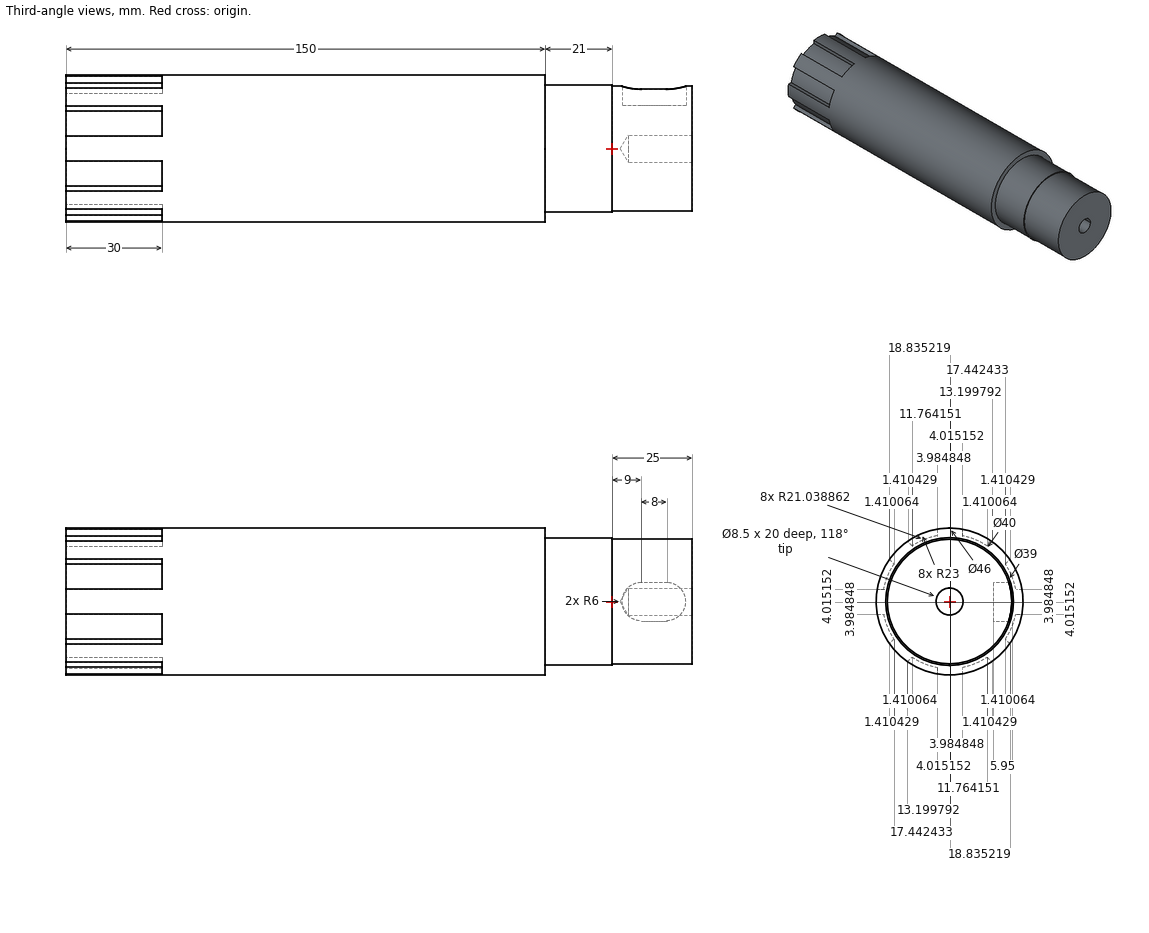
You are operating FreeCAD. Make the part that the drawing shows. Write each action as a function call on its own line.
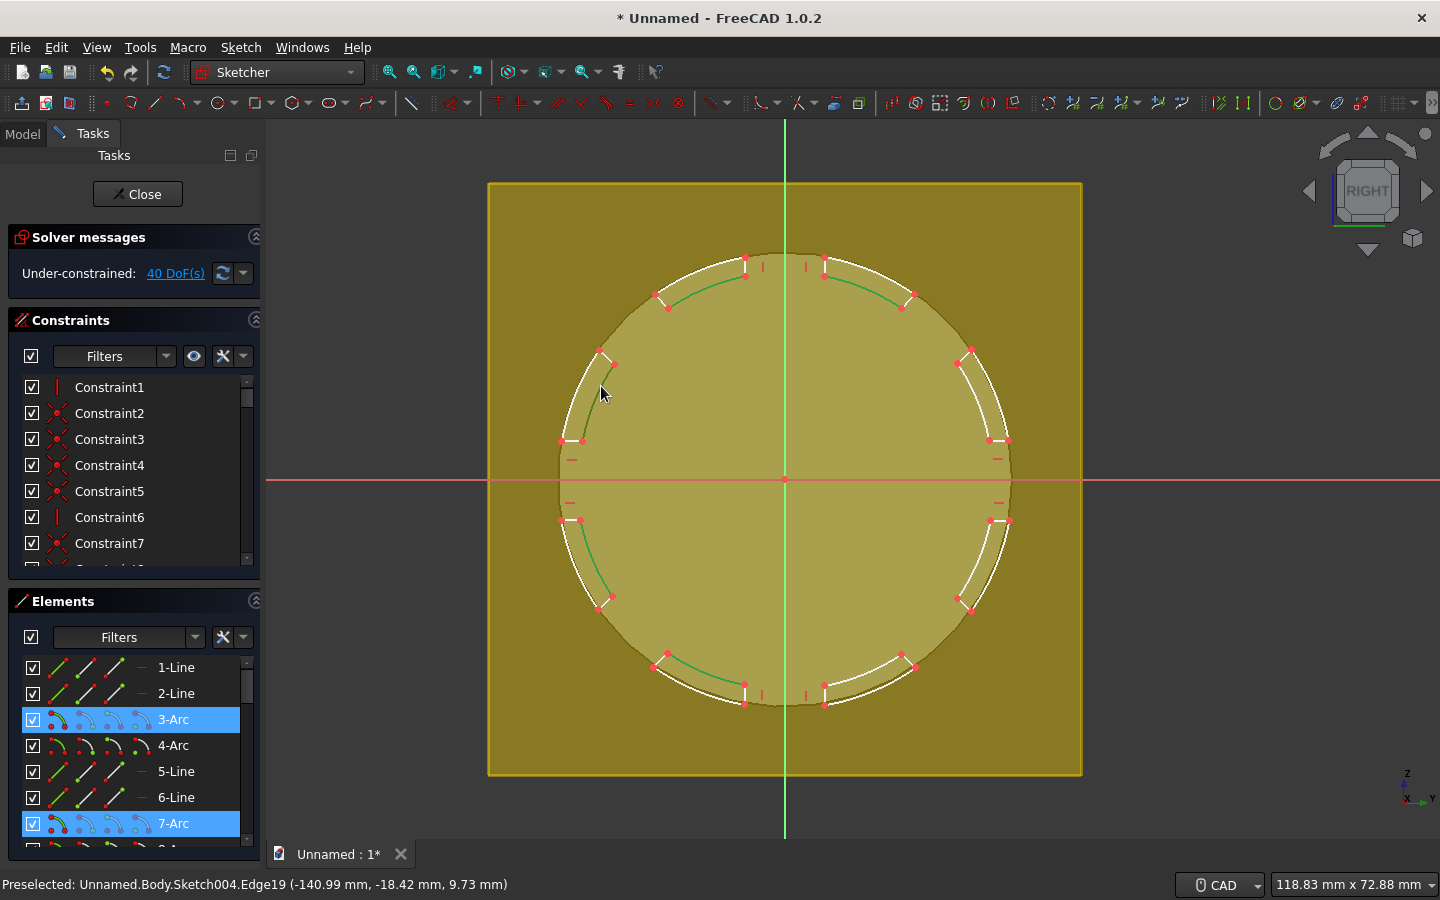
click(983, 416)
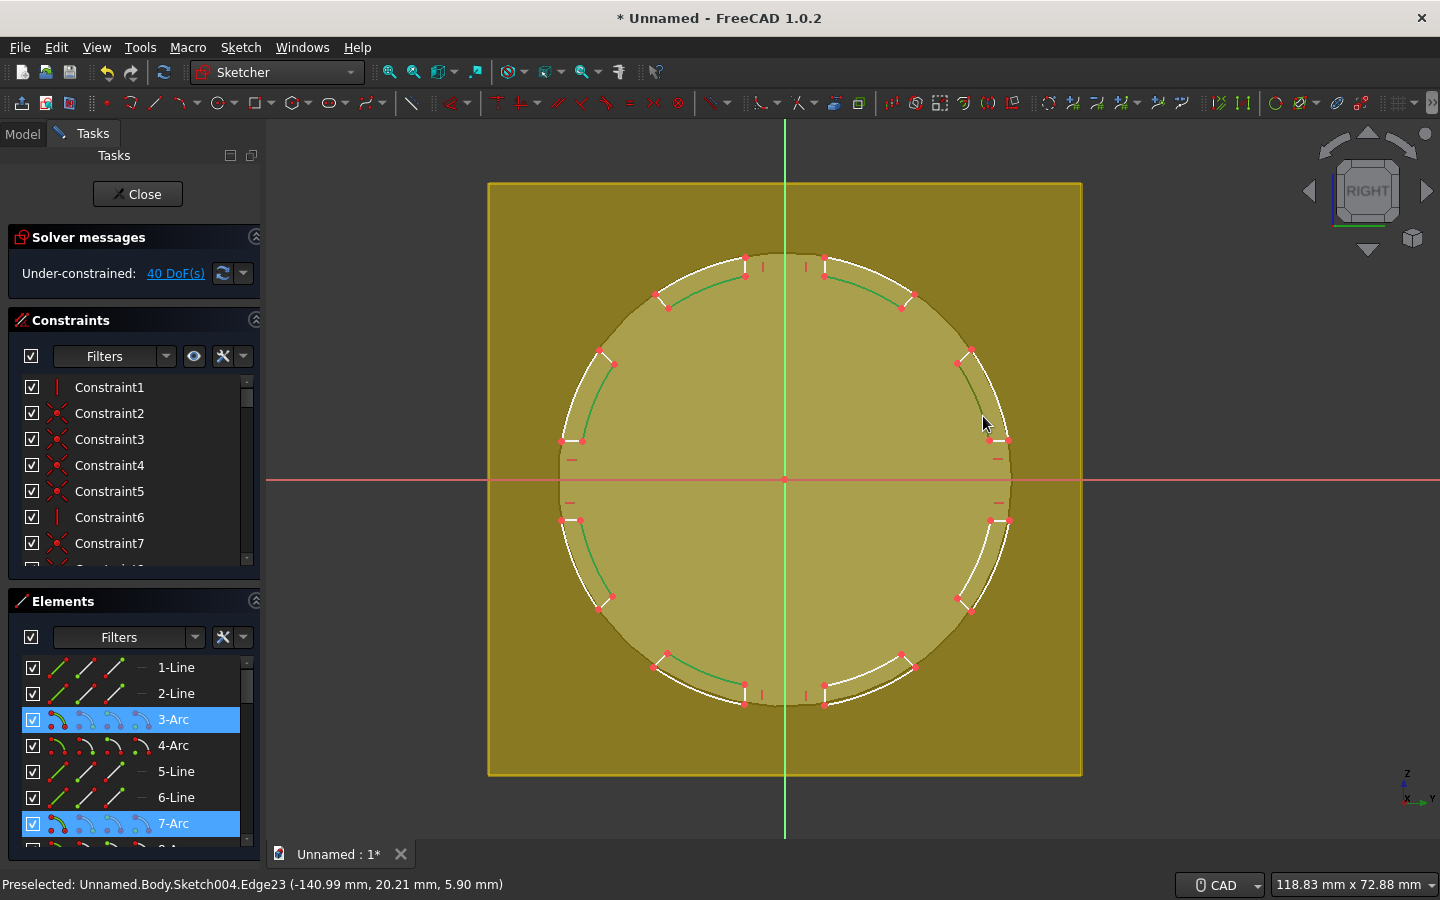
click(971, 576)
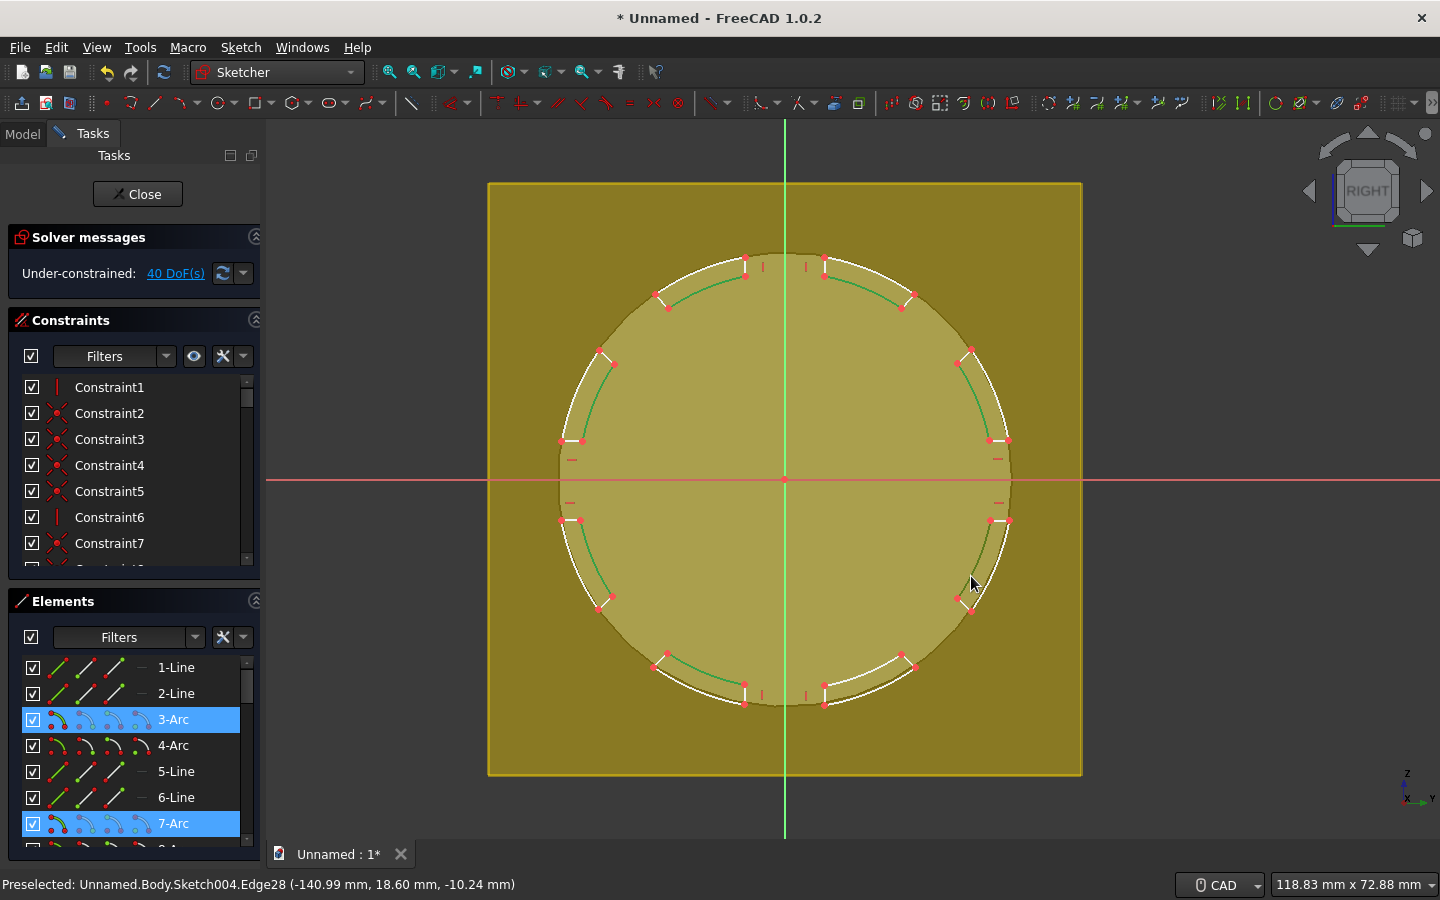
click(849, 680)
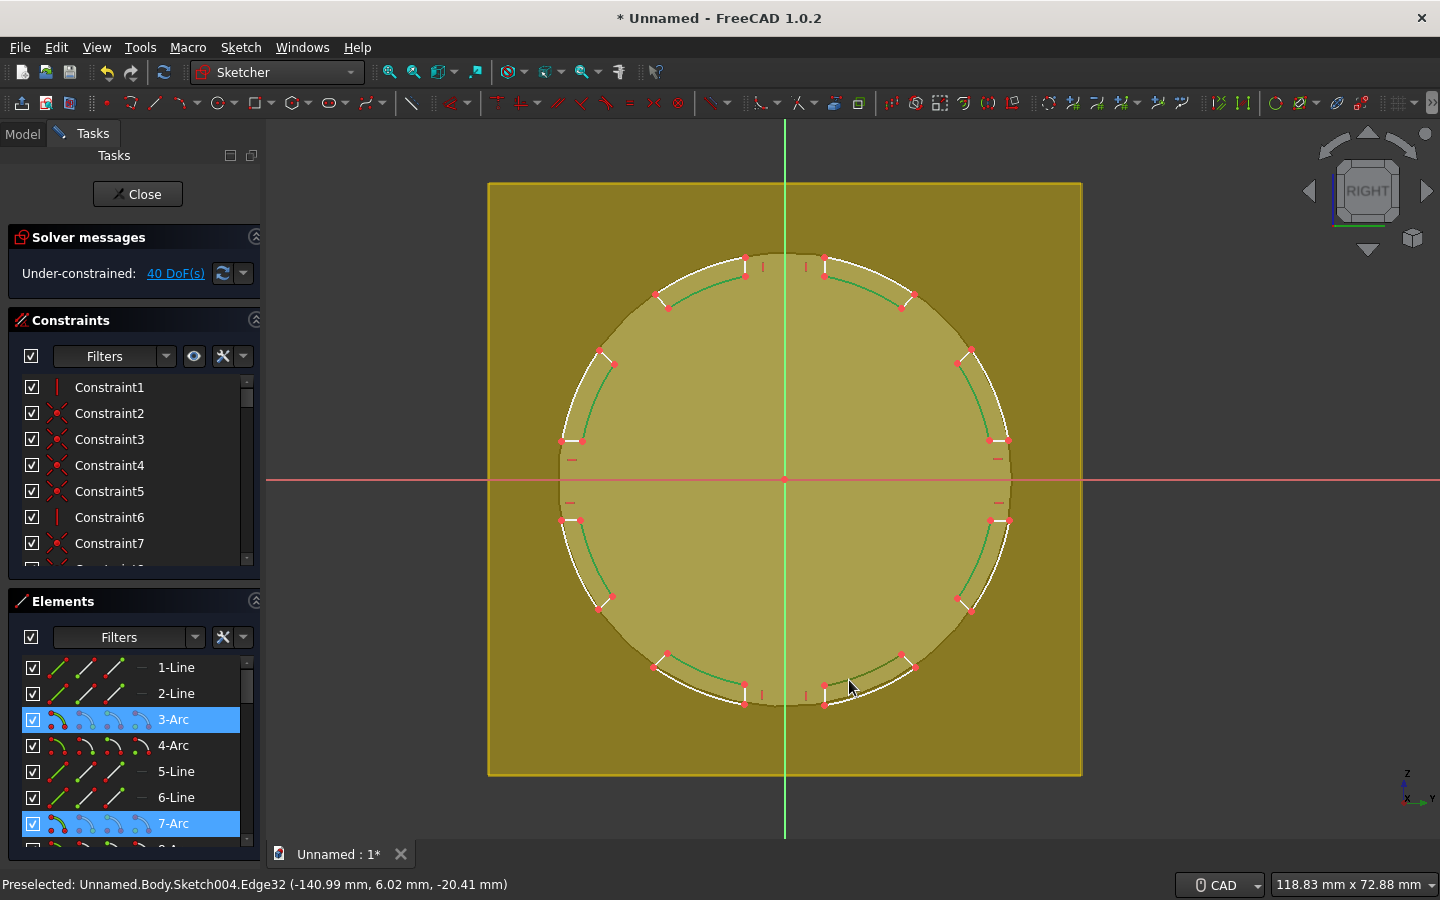
click(630, 104)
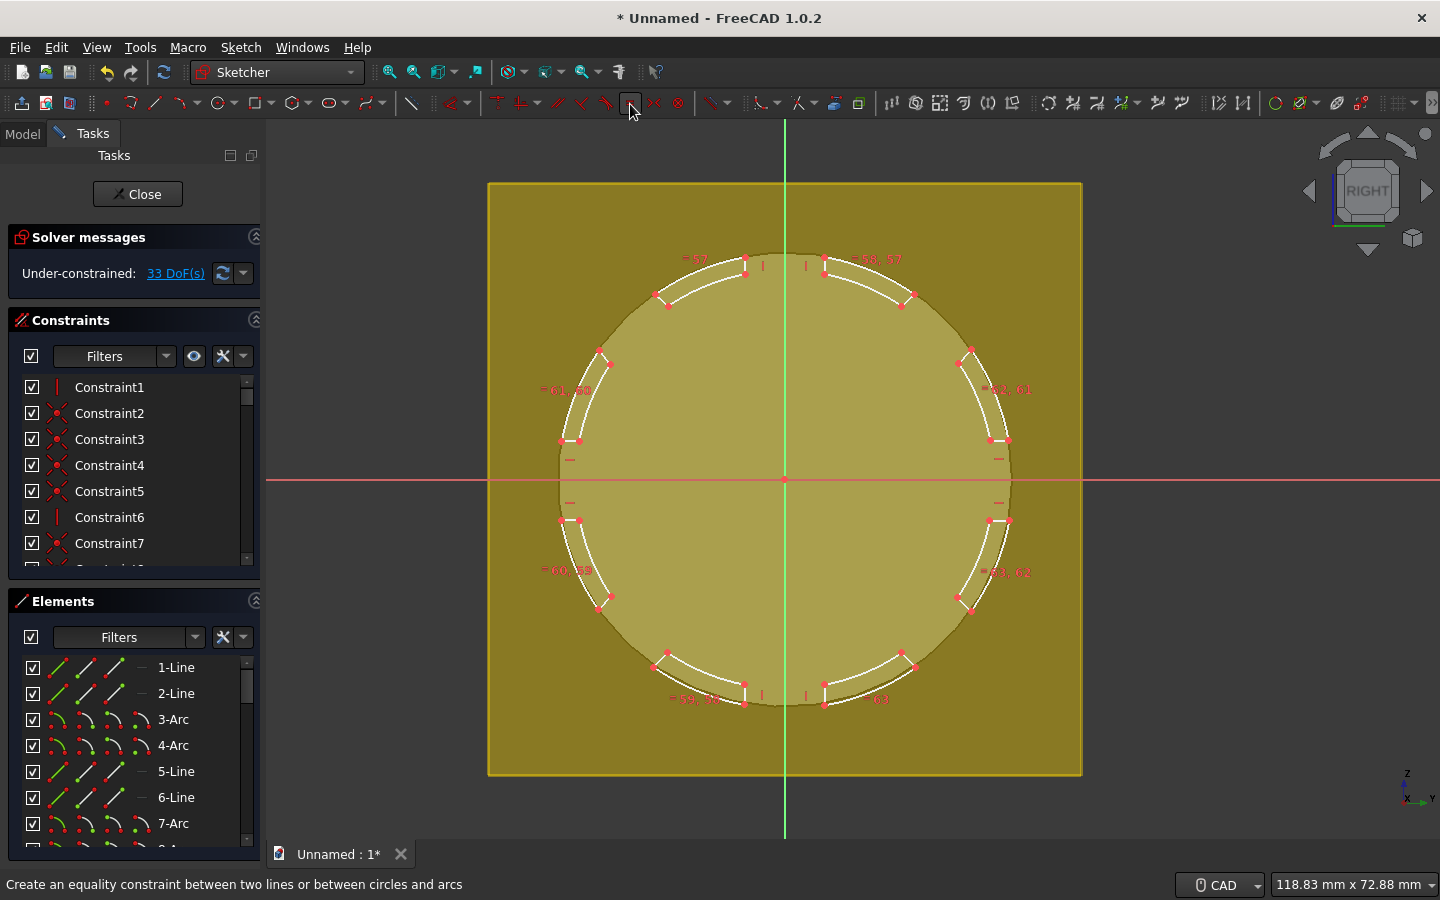
click(717, 264)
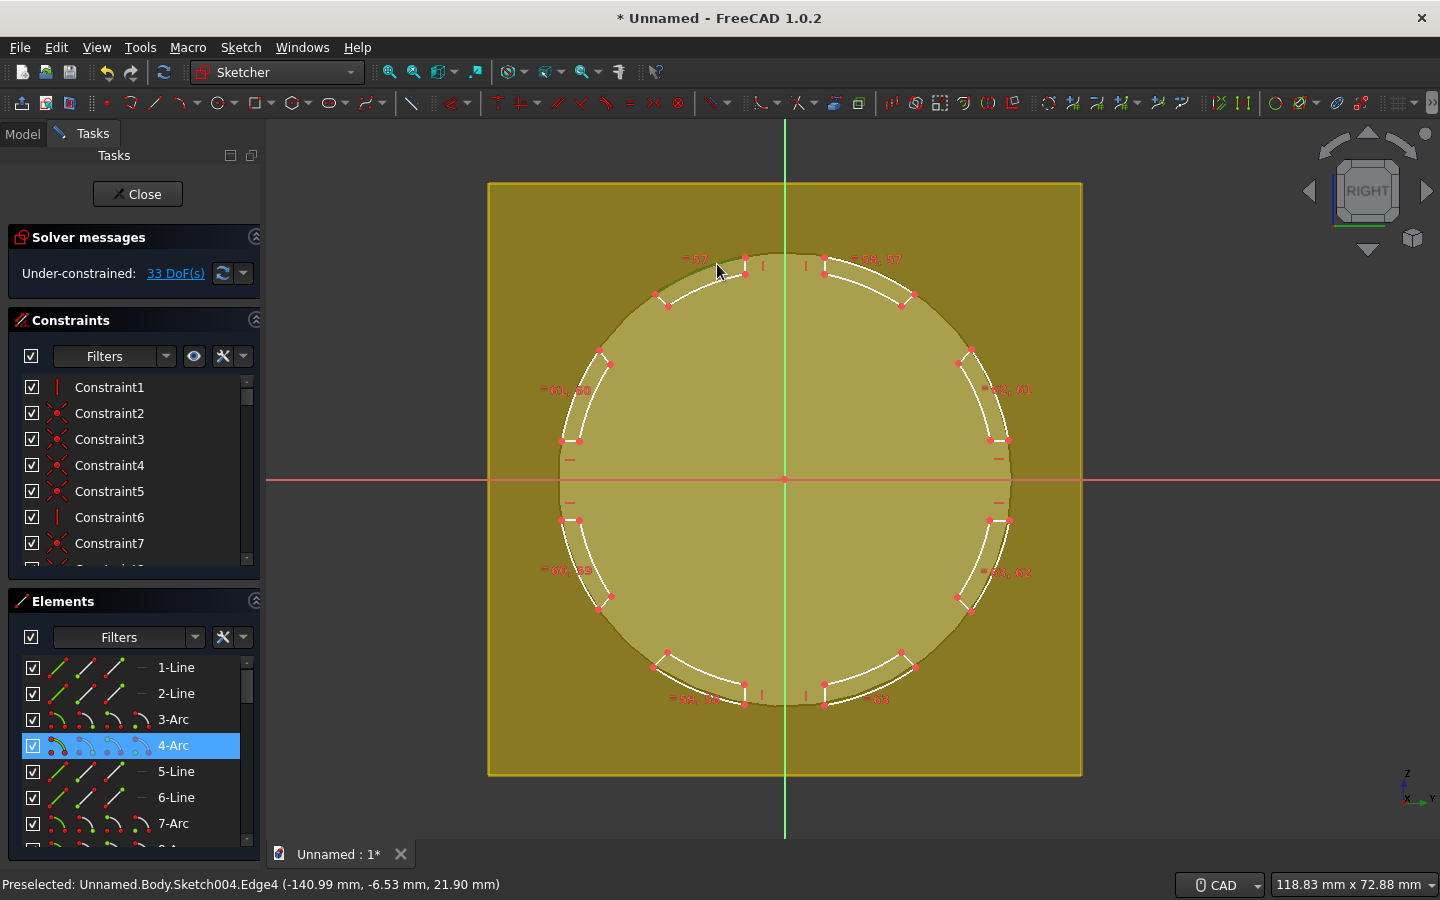
click(890, 279)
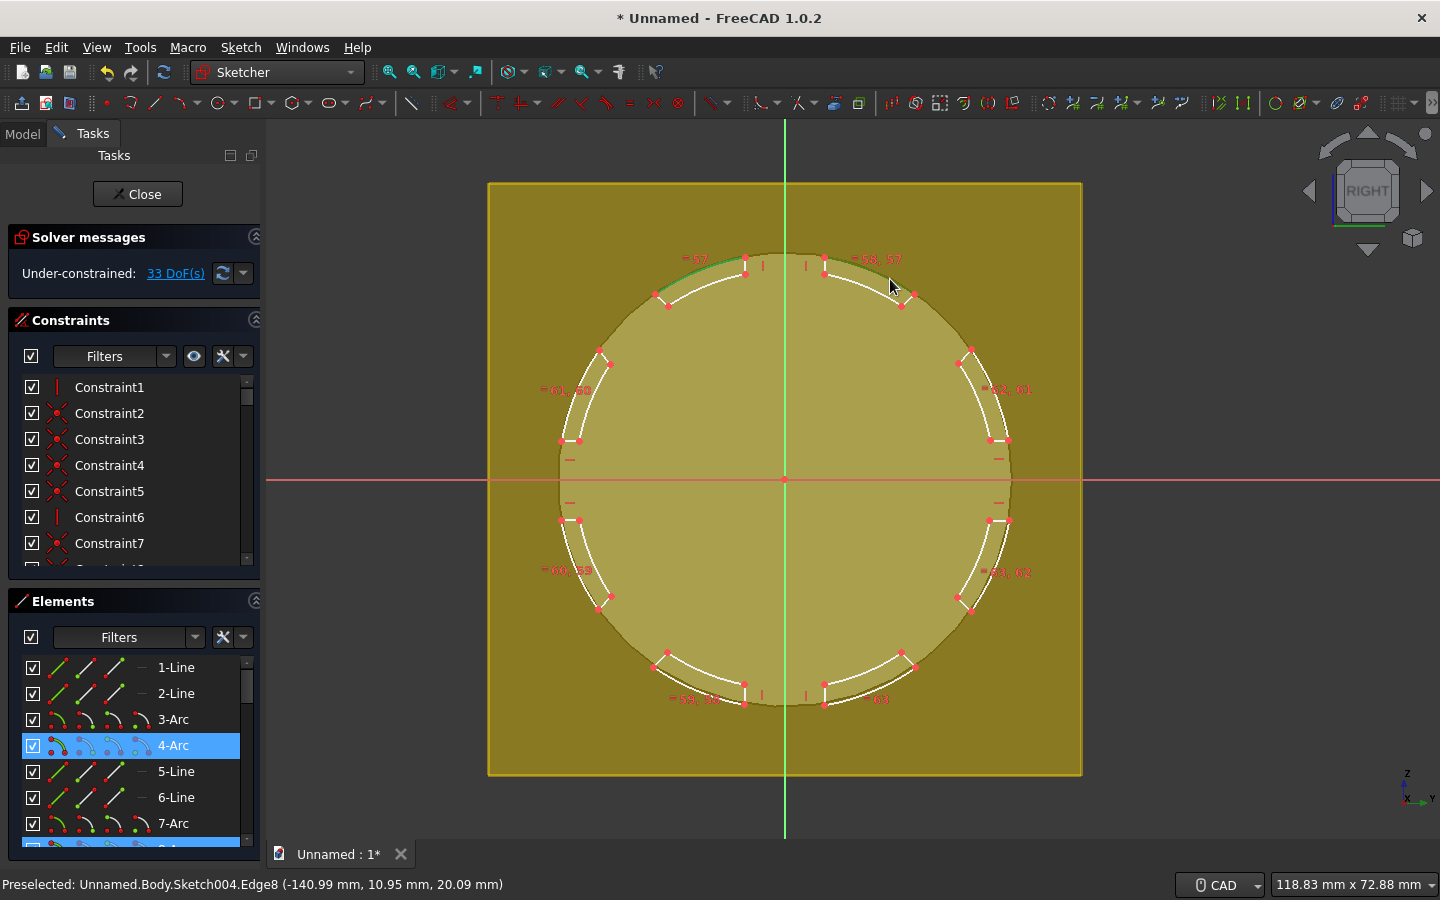
click(679, 683)